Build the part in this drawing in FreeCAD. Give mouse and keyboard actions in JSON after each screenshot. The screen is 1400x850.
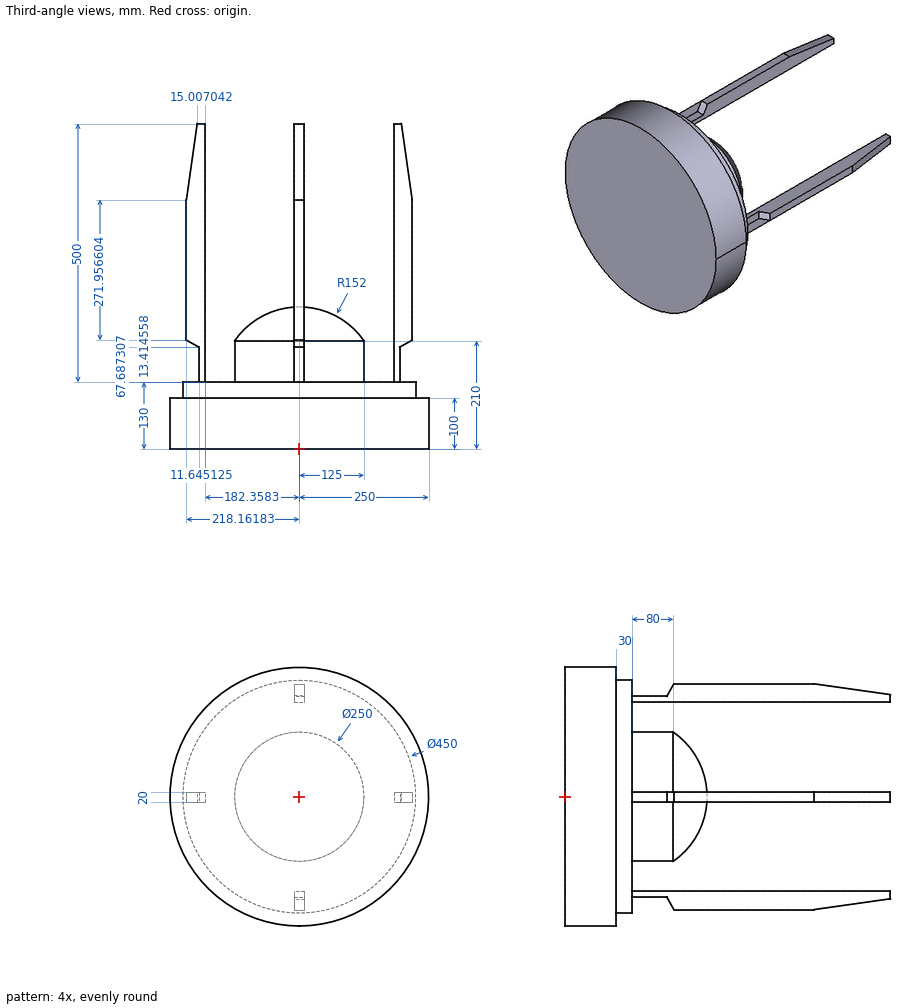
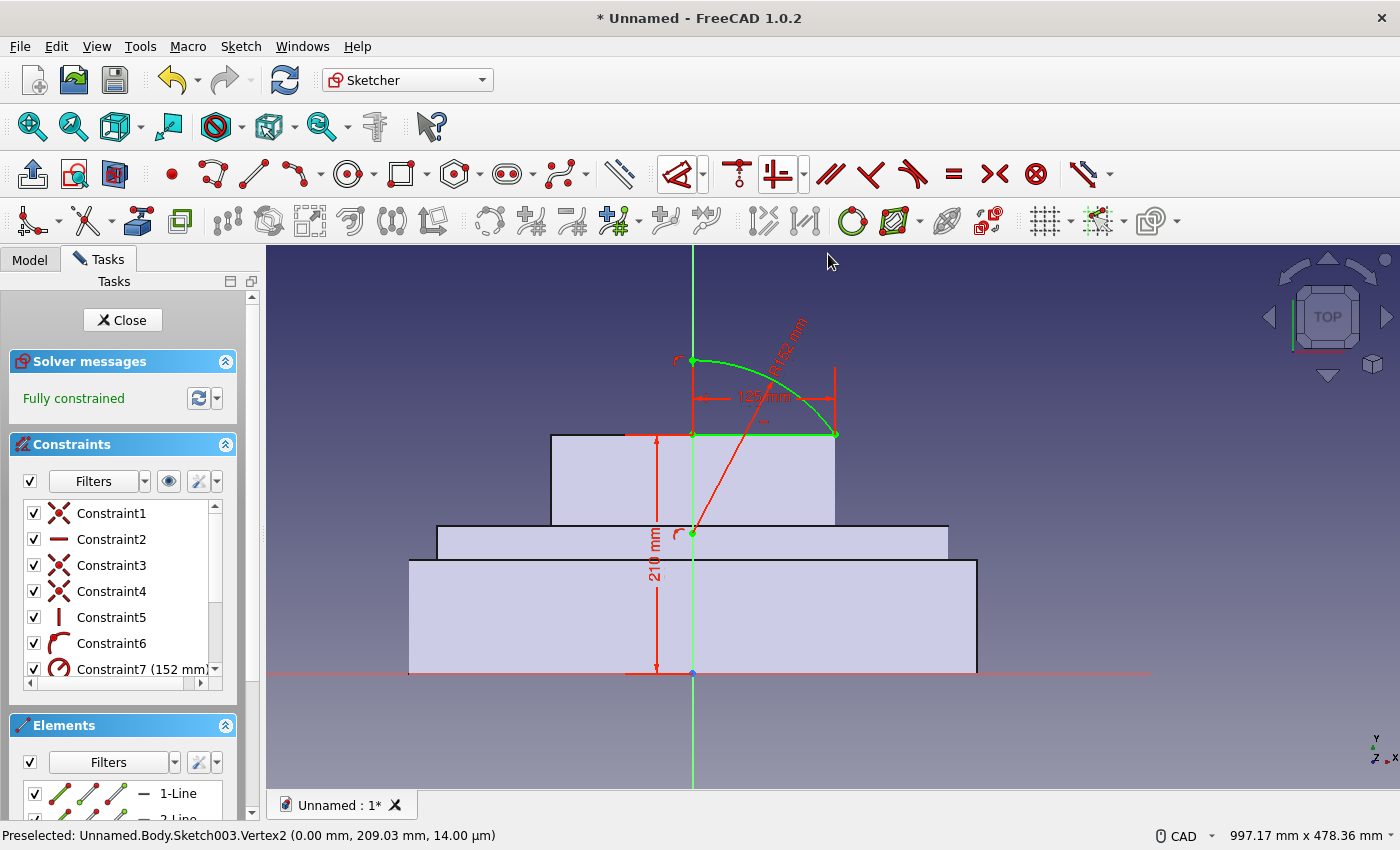
{"action": "left_click", "coordinate": [123, 320]}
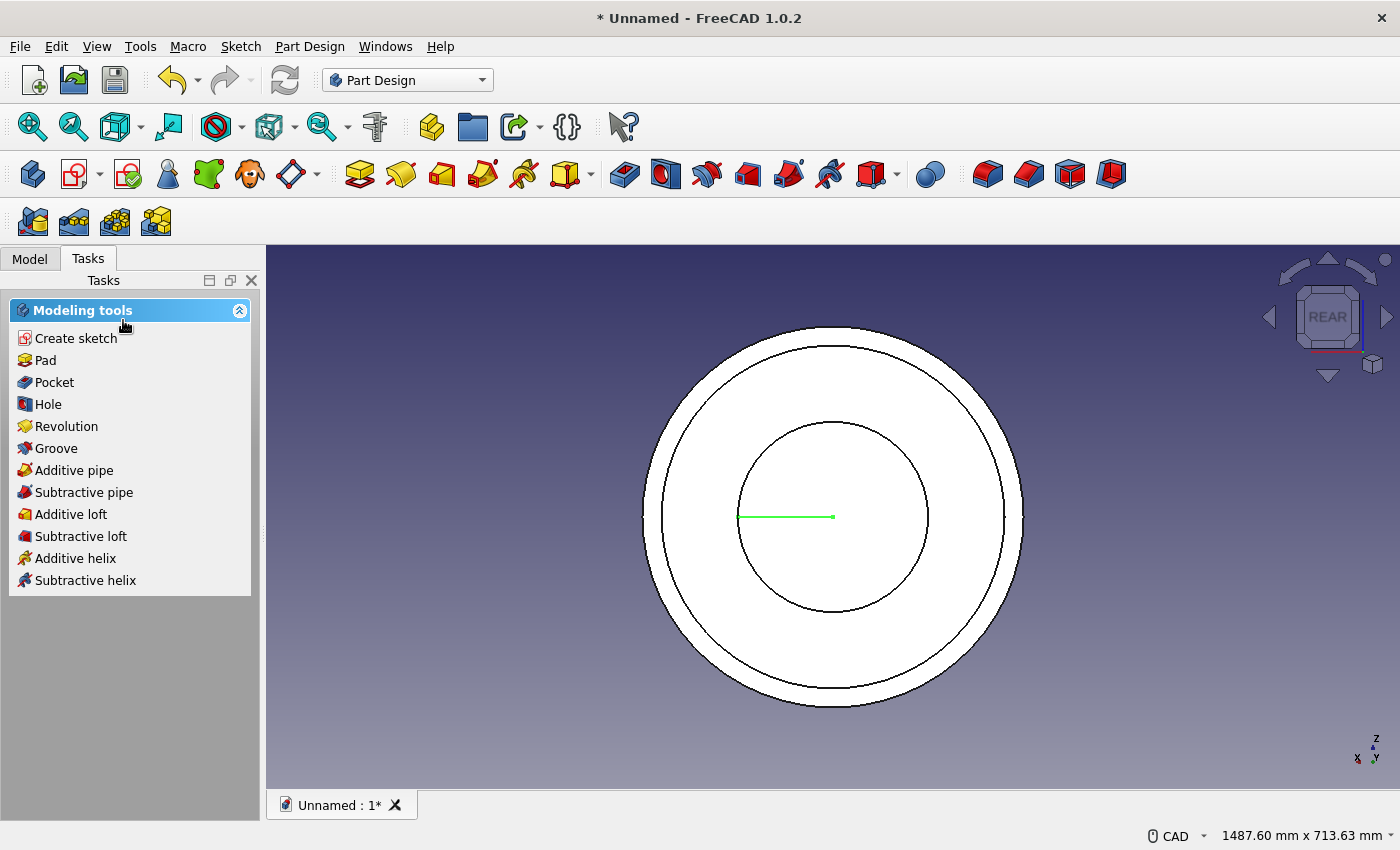
{"action": "left_click", "coordinate": [401, 174]}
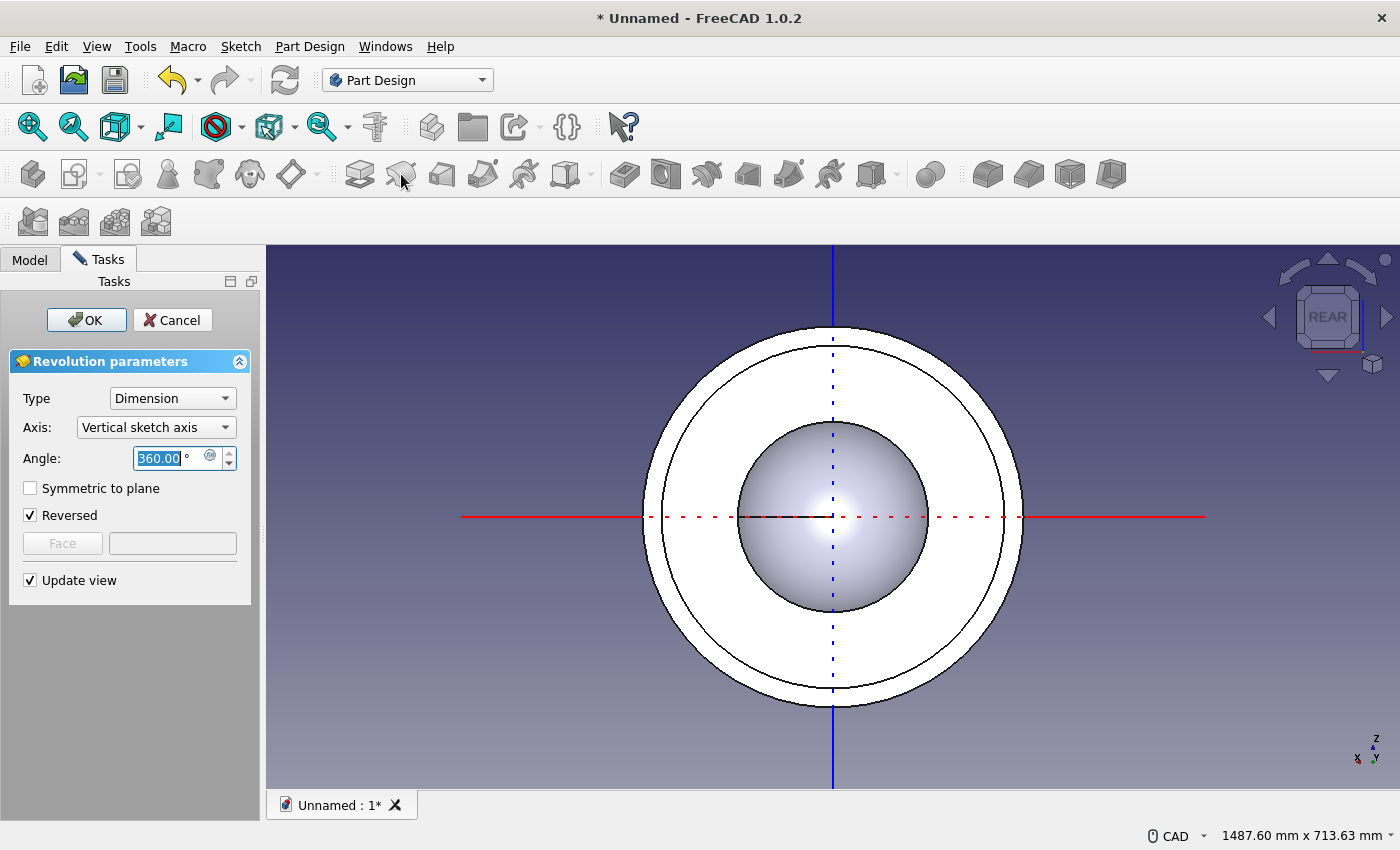
{"action": "left_click", "coordinate": [87, 320]}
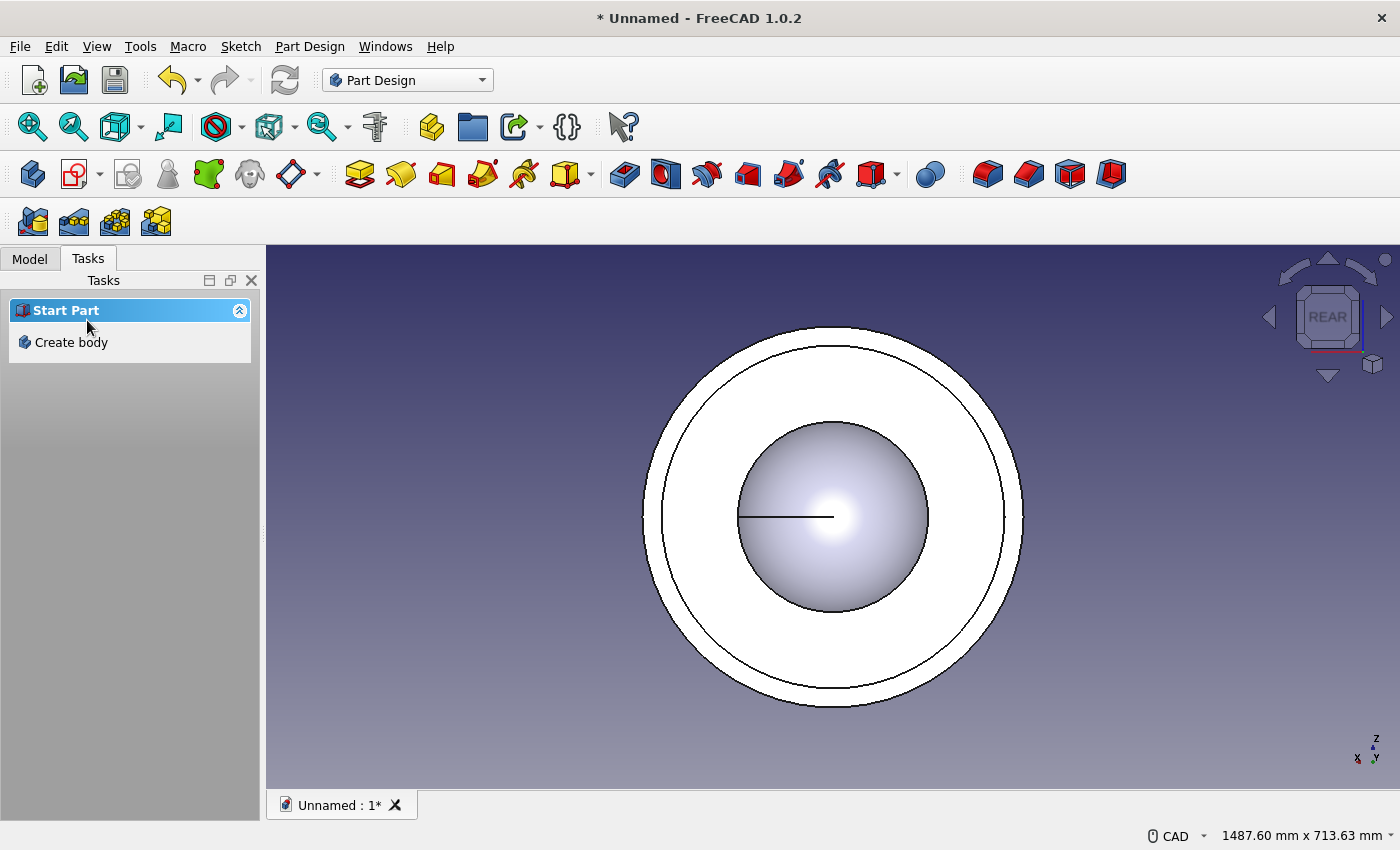
{"action": "left_click", "coordinate": [74, 174]}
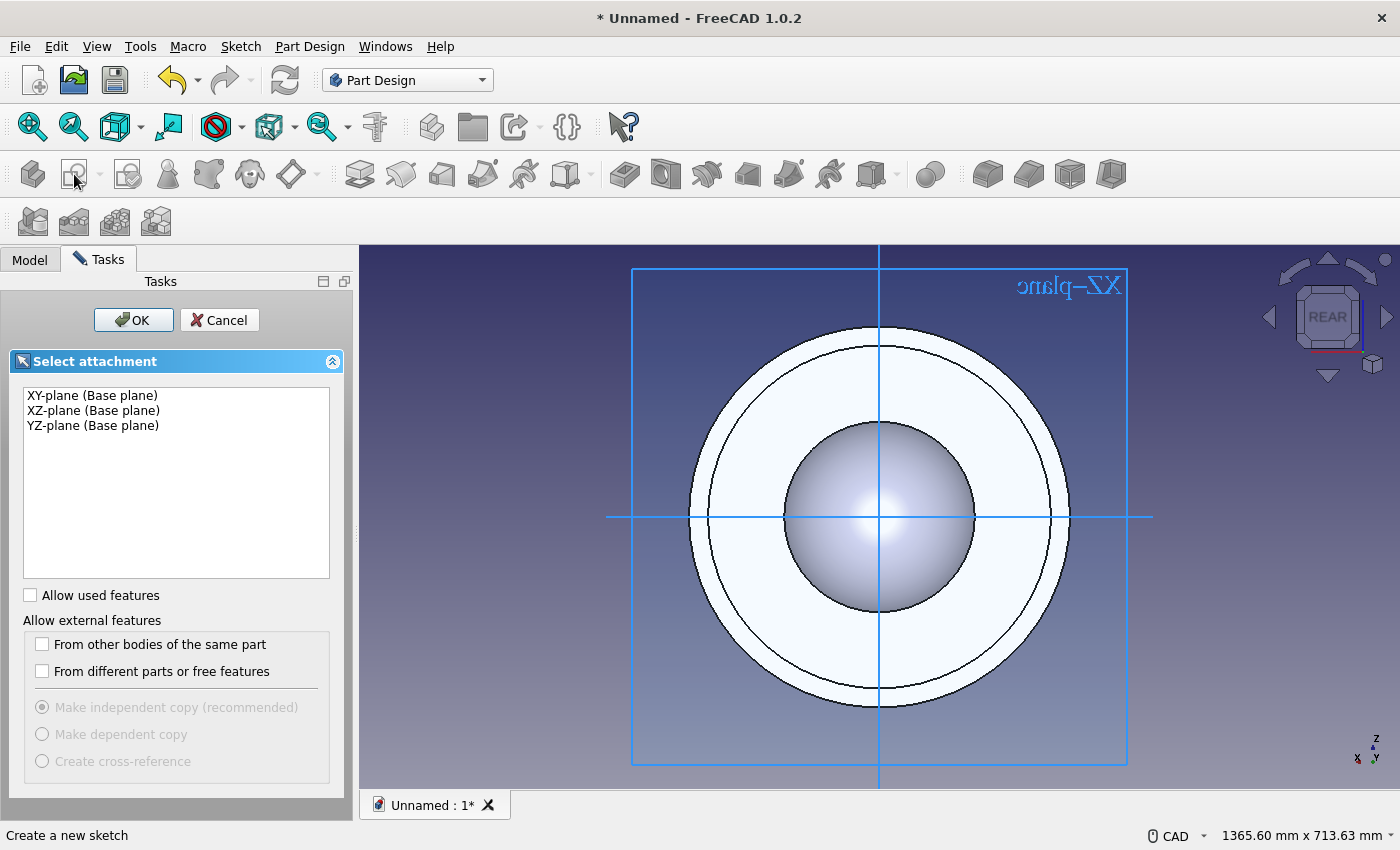
{"action": "left_click", "coordinate": [84, 396]}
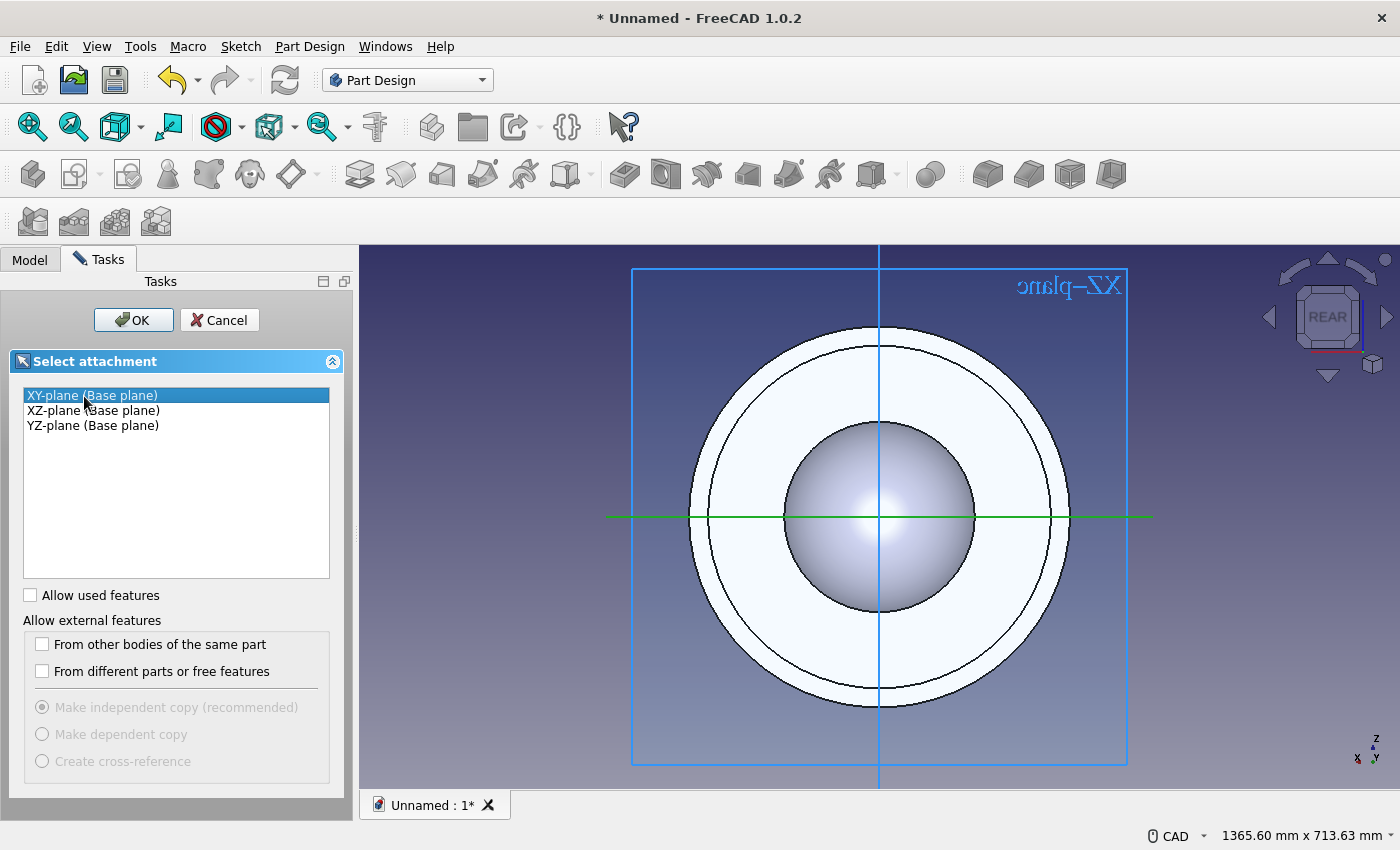
{"action": "left_click", "coordinate": [134, 320]}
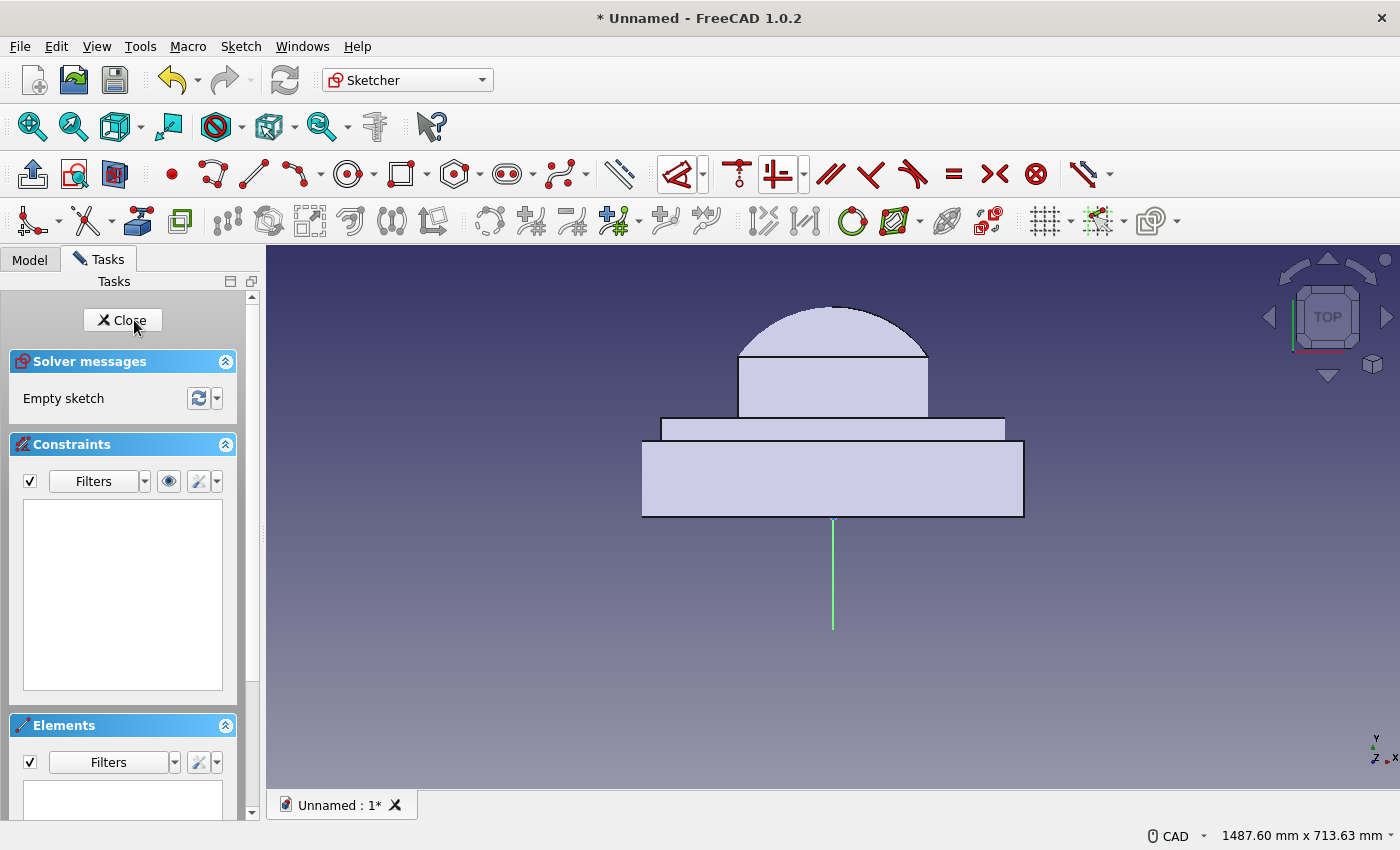
{"action": "left_click", "coordinate": [115, 174]}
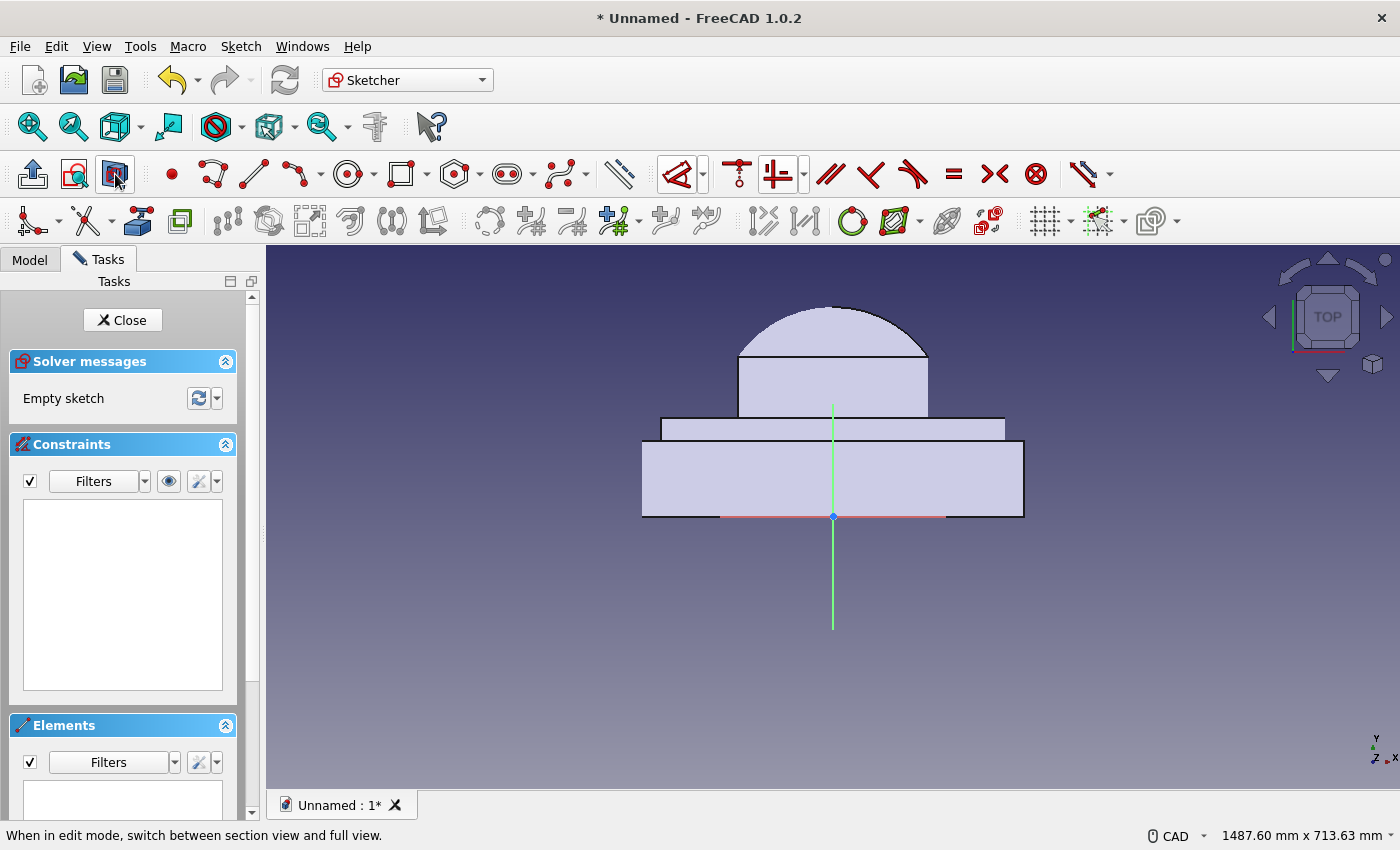
{"action": "scroll", "coordinate": [782, 761], "scroll_direction": "down", "scroll_amount": 3}